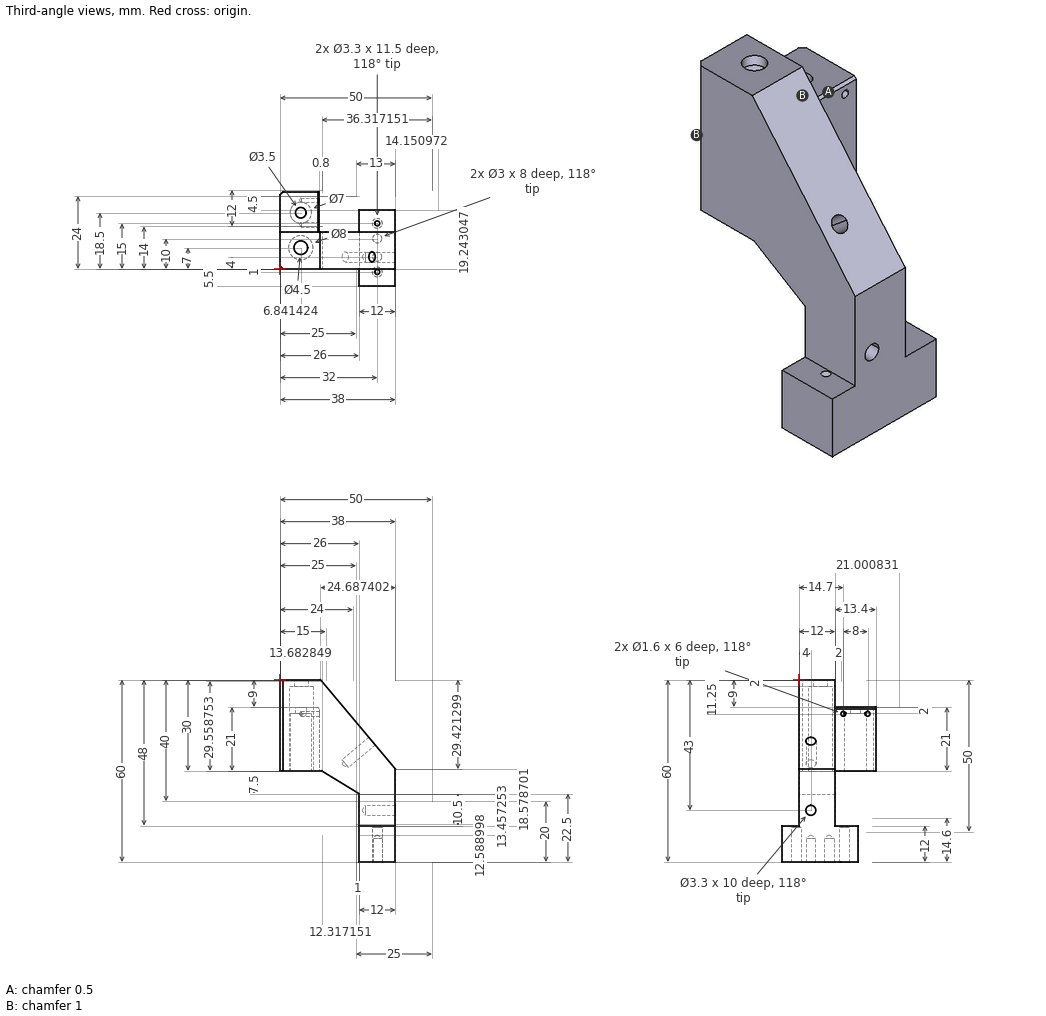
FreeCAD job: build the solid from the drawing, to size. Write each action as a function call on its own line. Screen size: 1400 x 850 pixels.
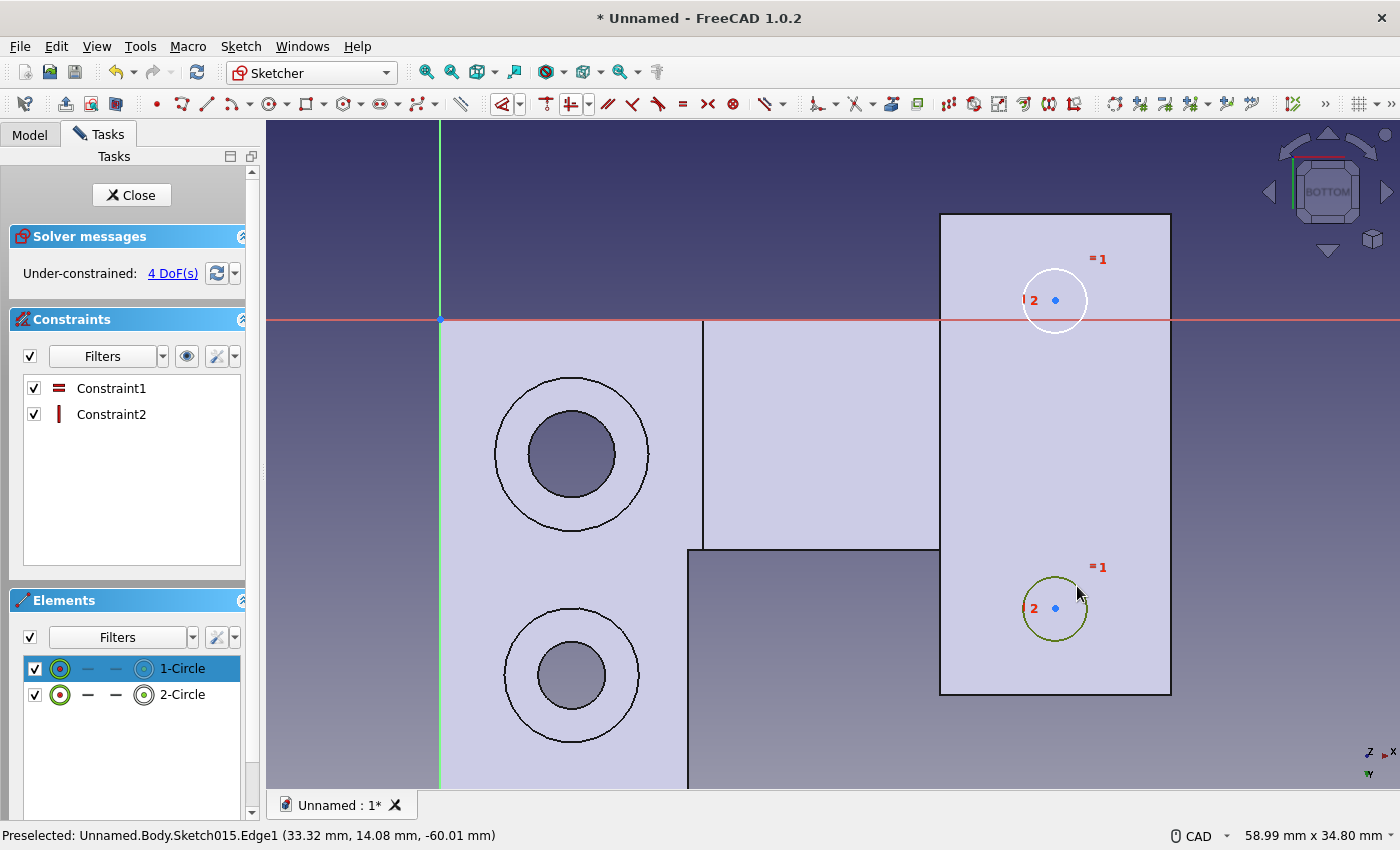
key(k)
key(o)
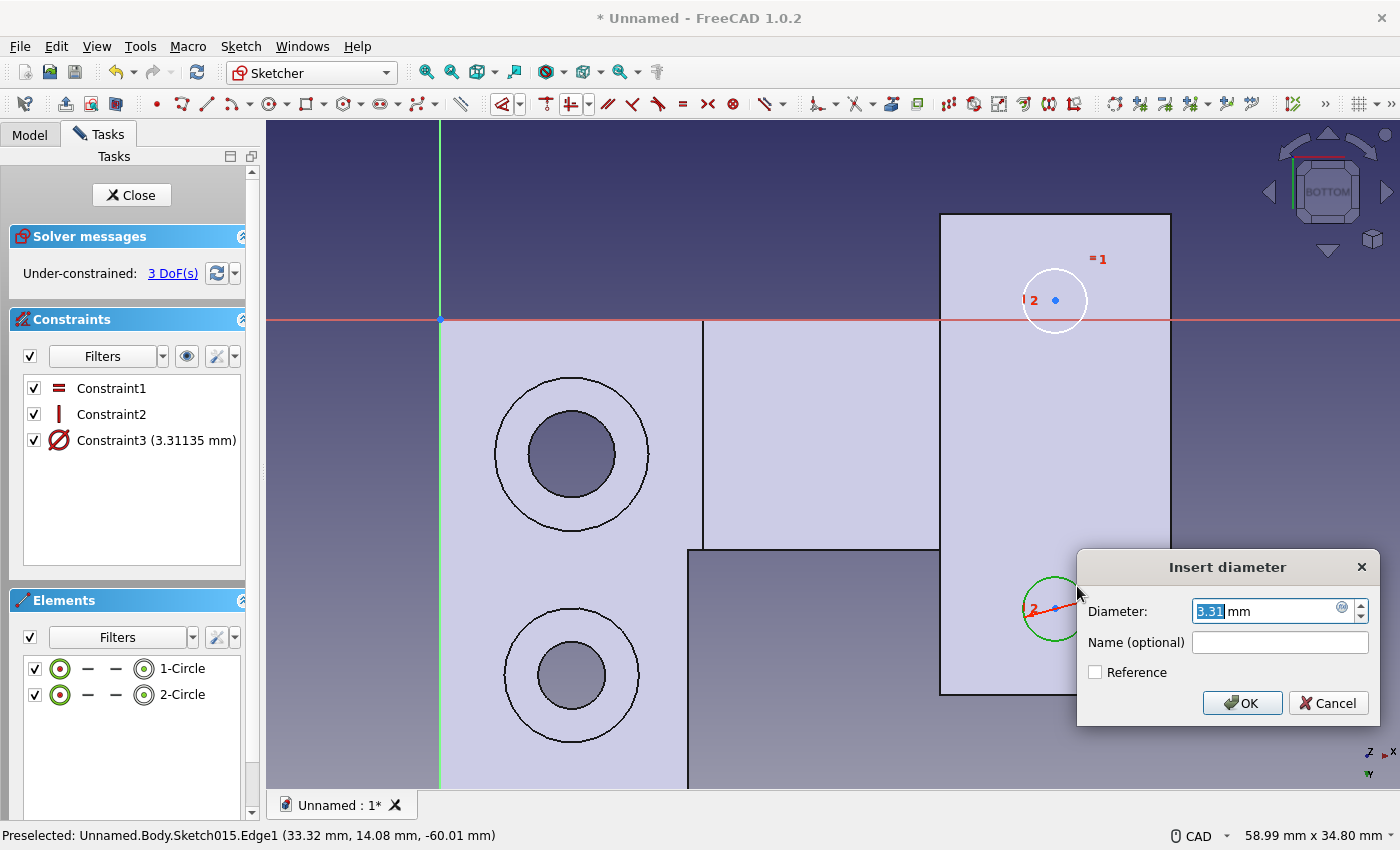
text(3.3)
key(Return)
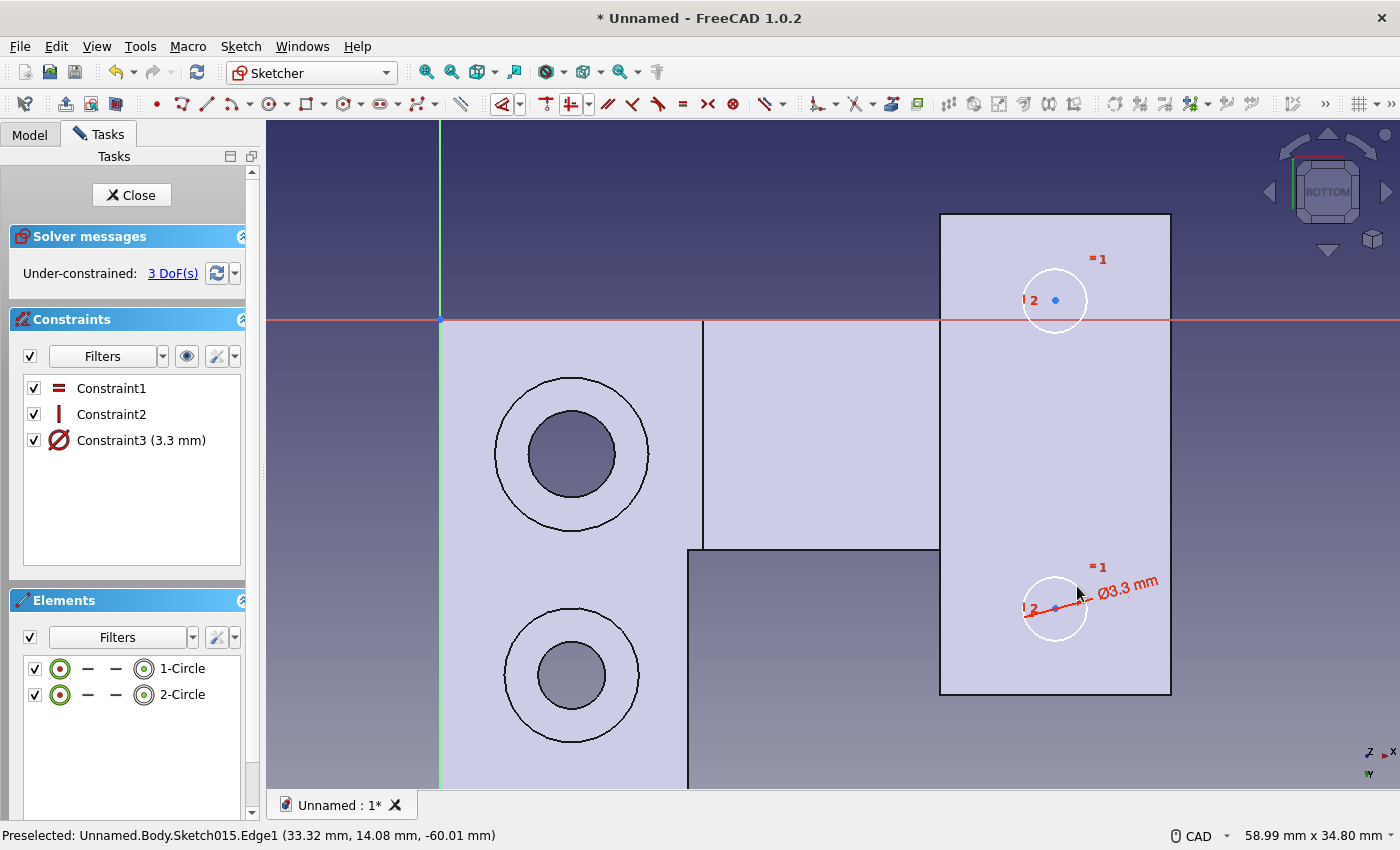
scroll(1055, 301, up, 4)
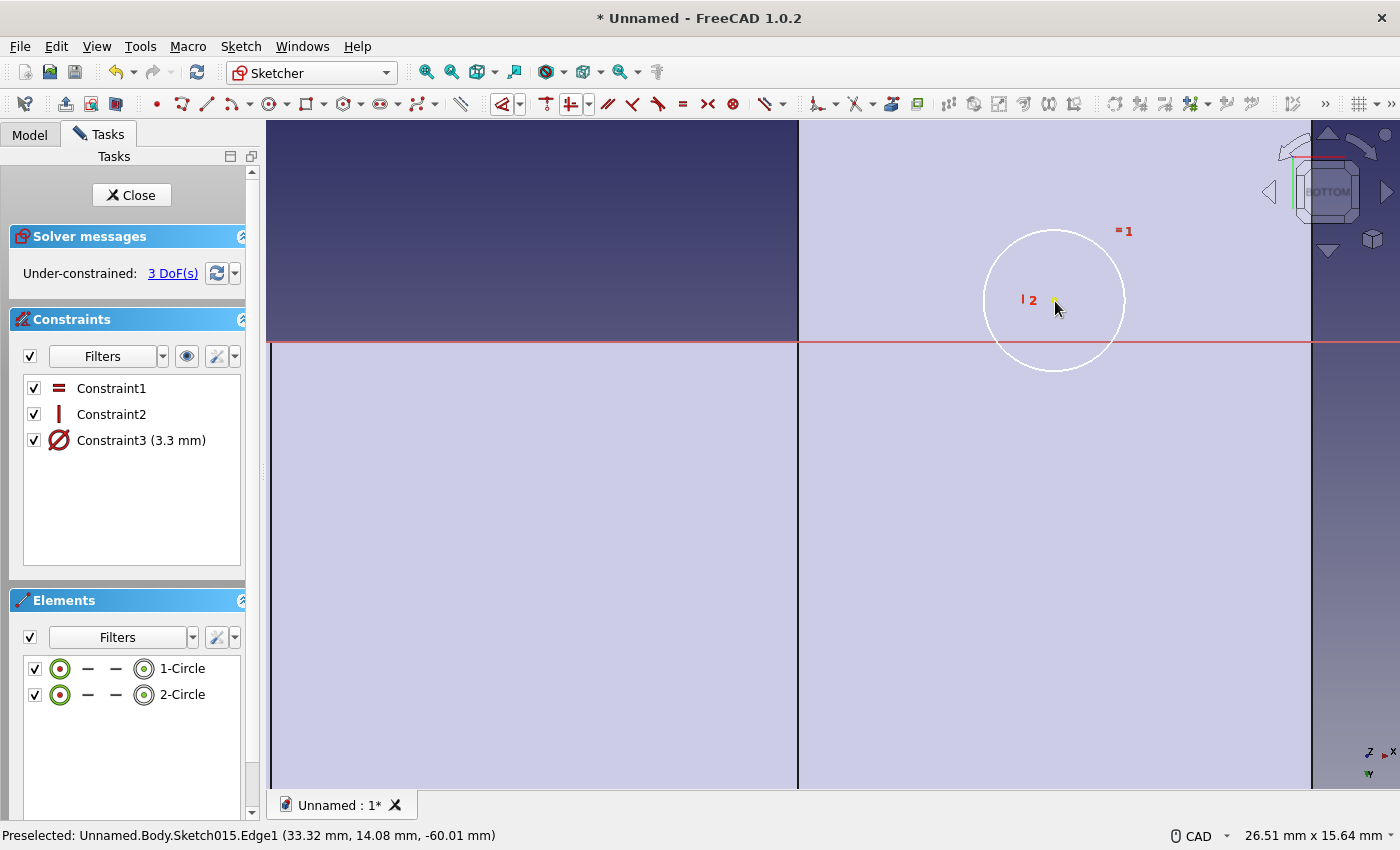
click(1054, 301)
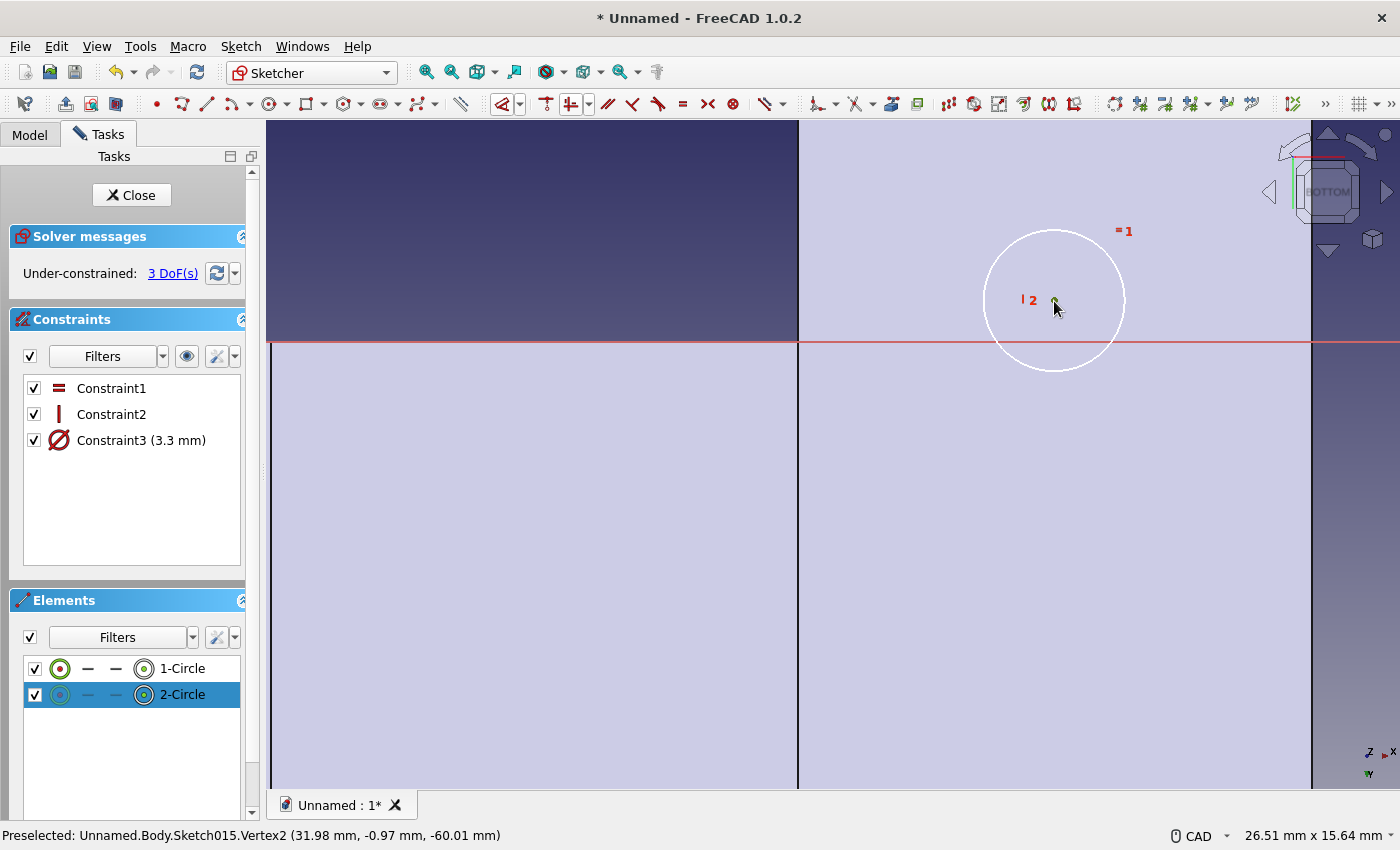
key(i)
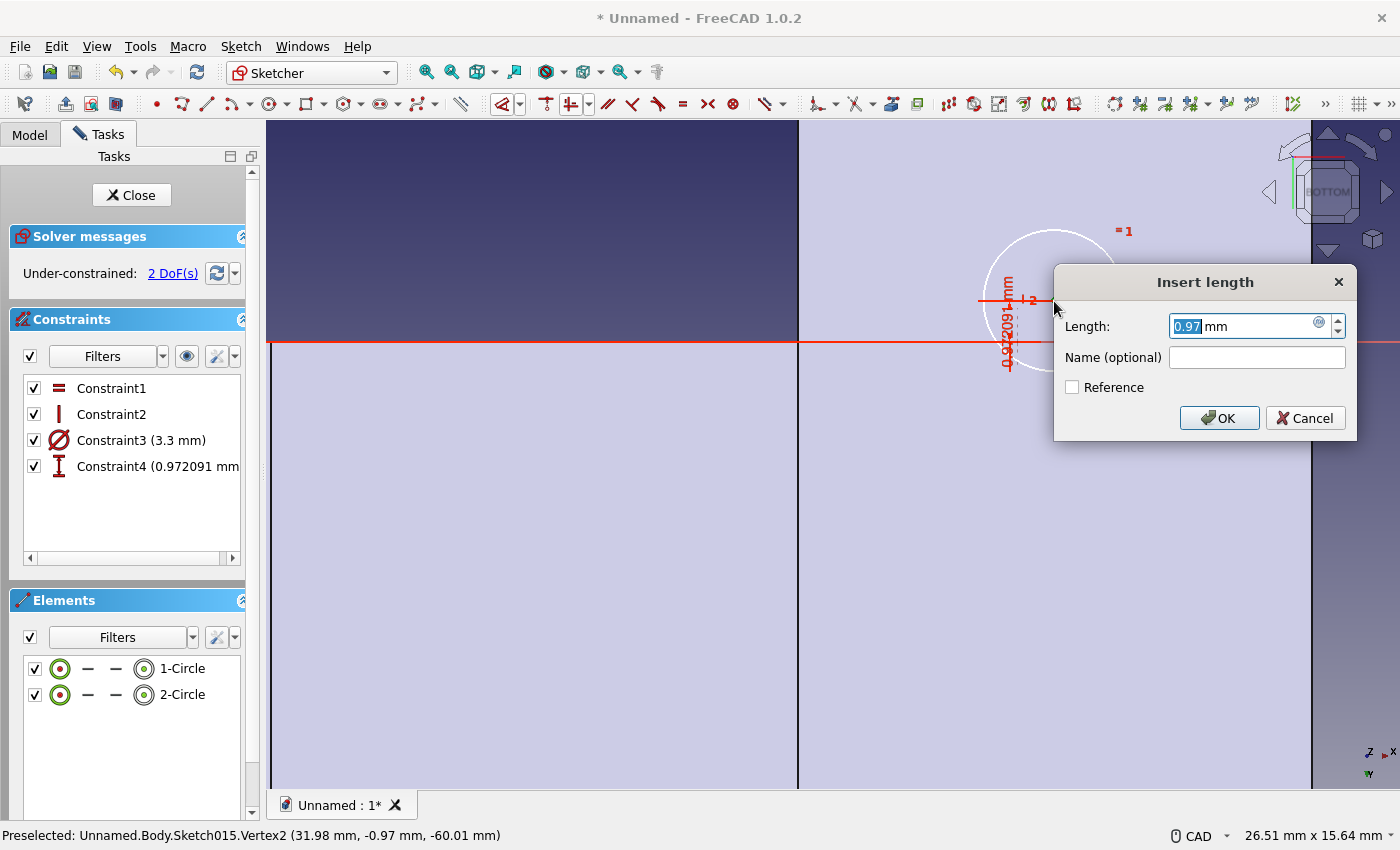
text(1)
key(Return)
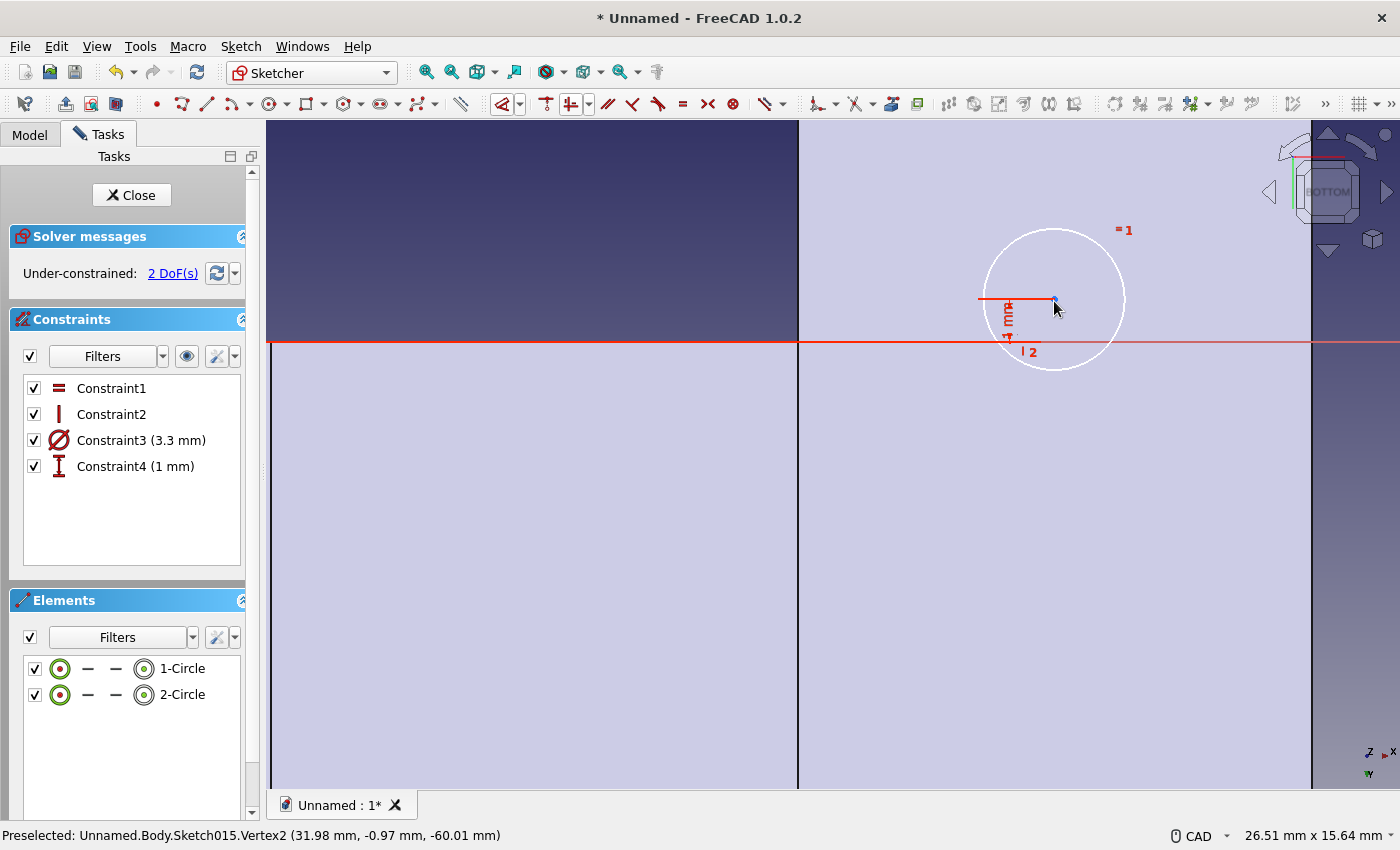
scroll(1057, 302, down, 4)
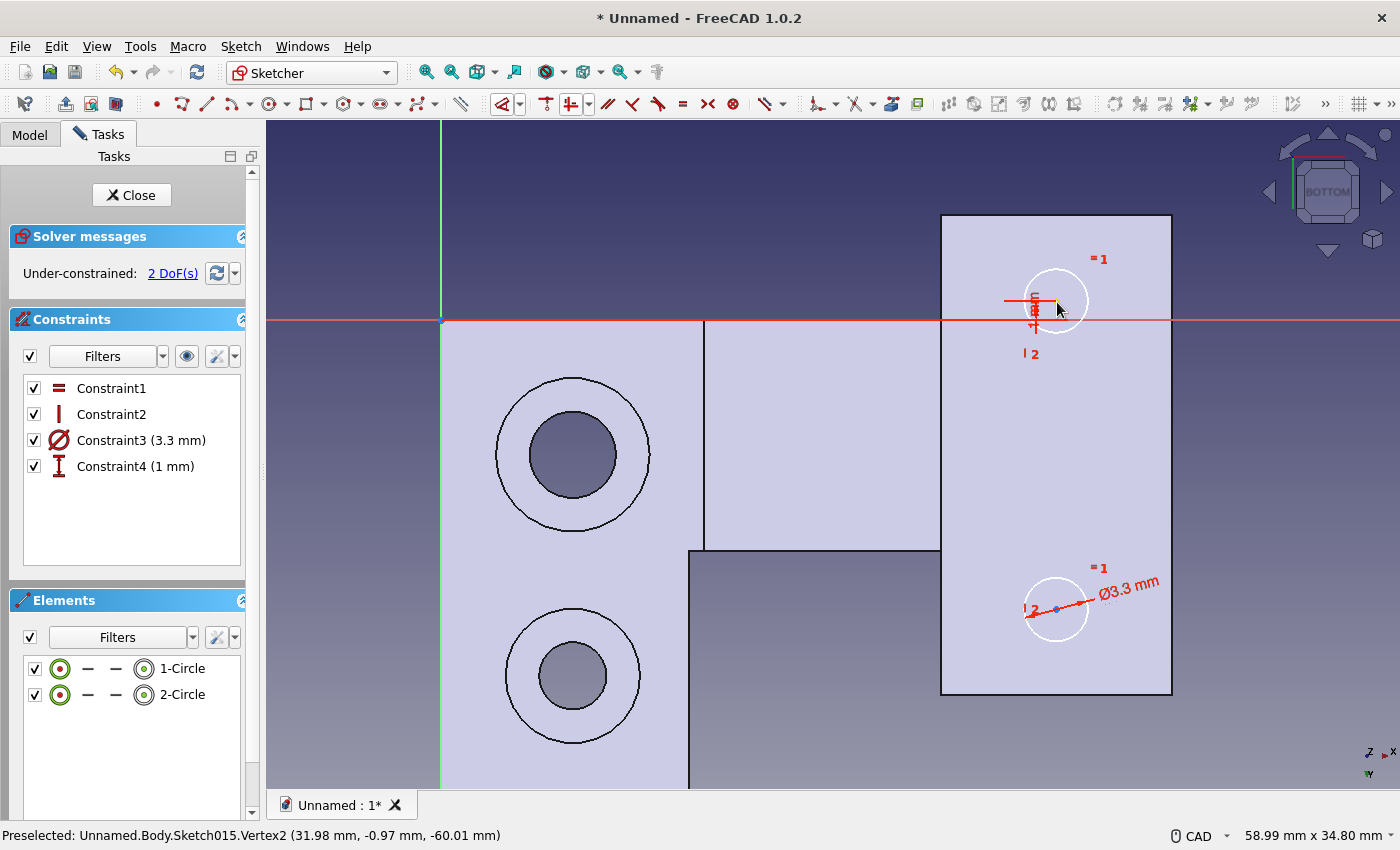
click(1056, 610)